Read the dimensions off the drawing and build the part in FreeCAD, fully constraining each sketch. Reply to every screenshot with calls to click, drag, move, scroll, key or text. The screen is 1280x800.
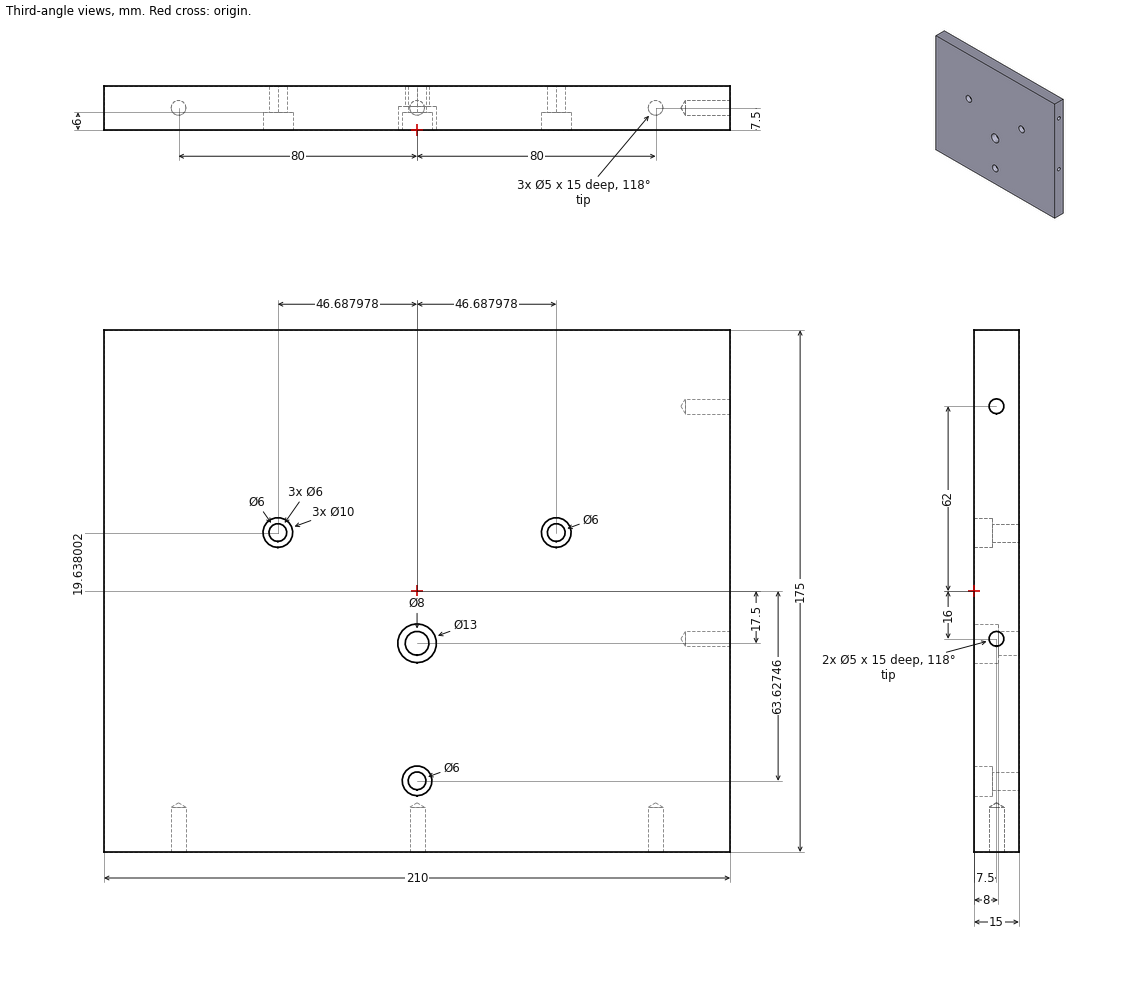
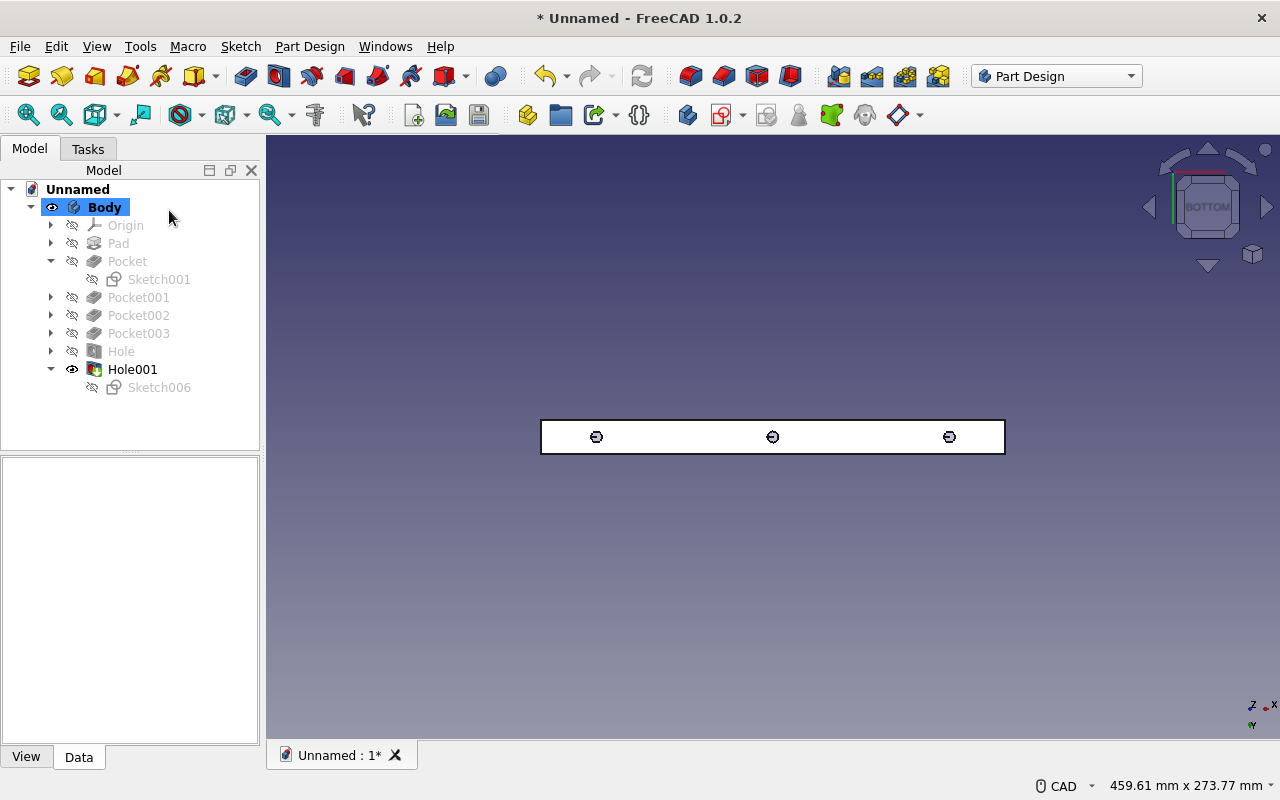
click(720, 116)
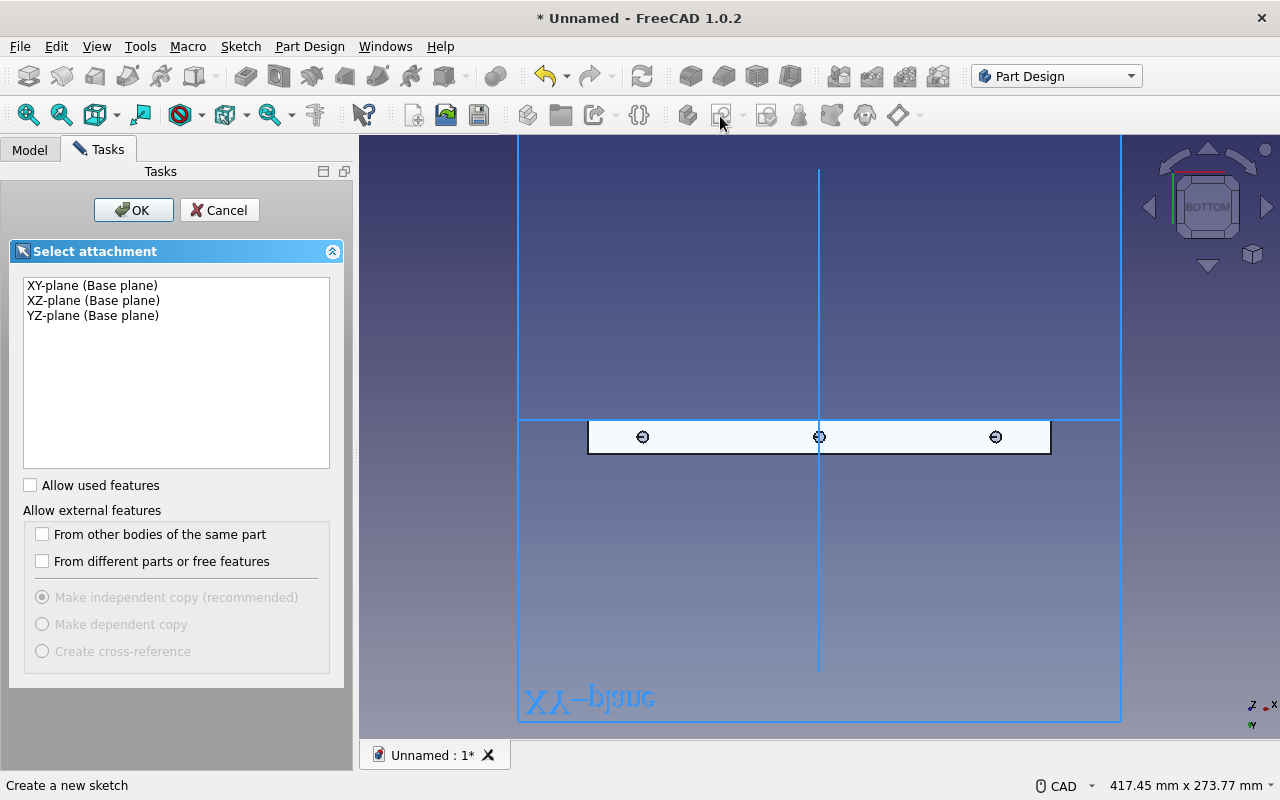
click(84, 300)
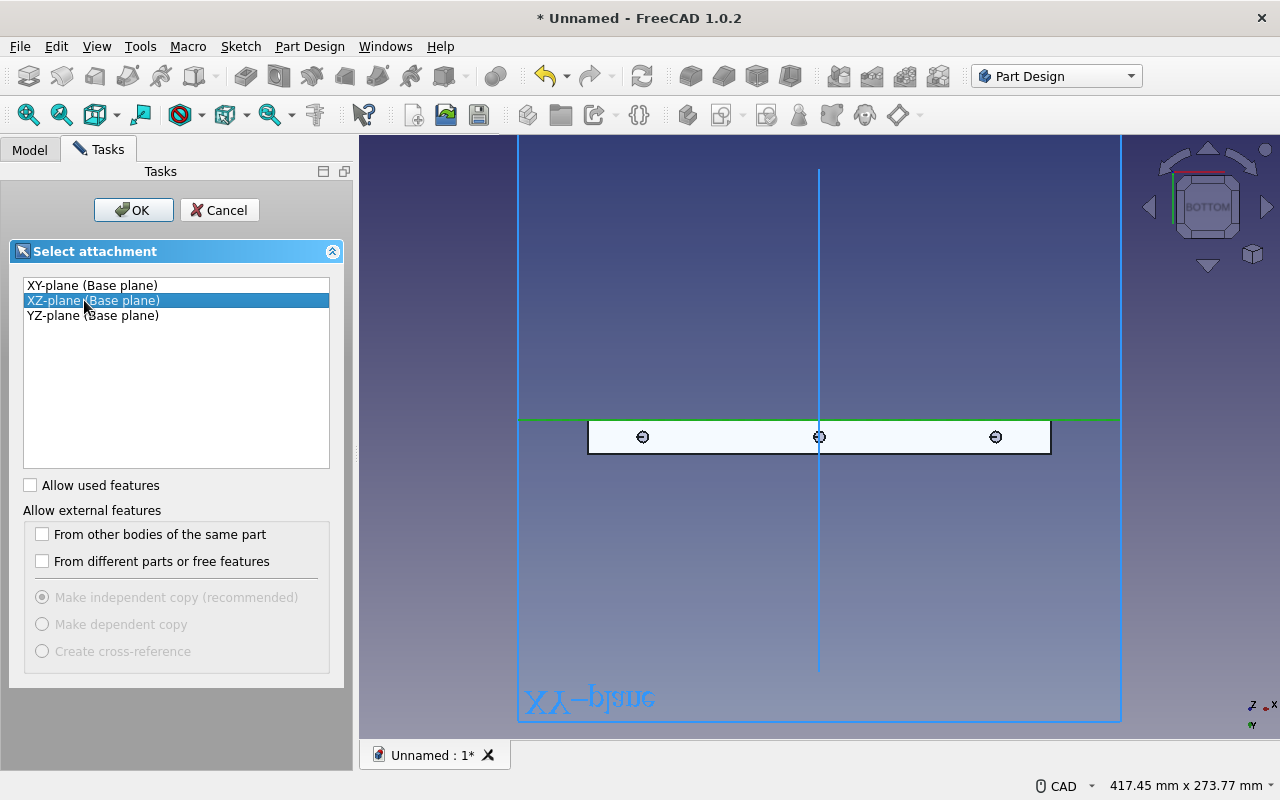
click(134, 210)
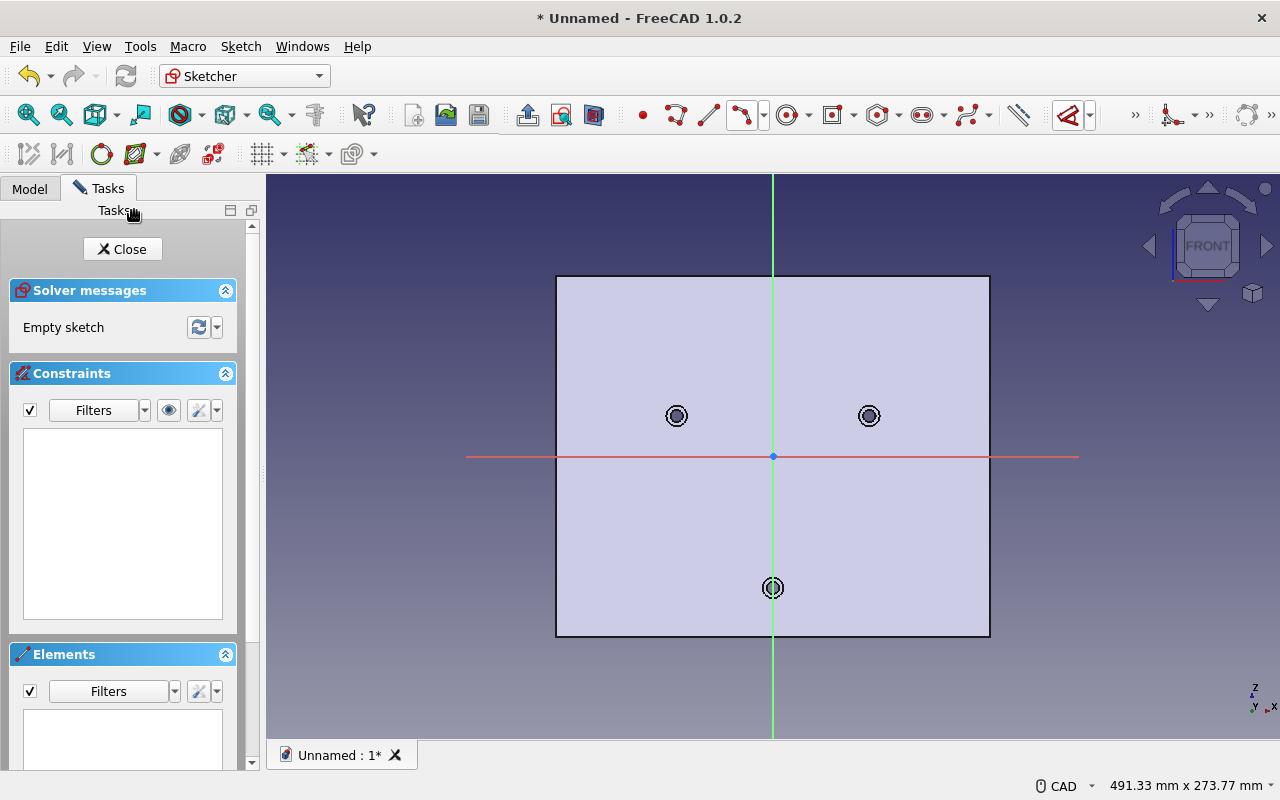
scroll(784, 485, up, 10)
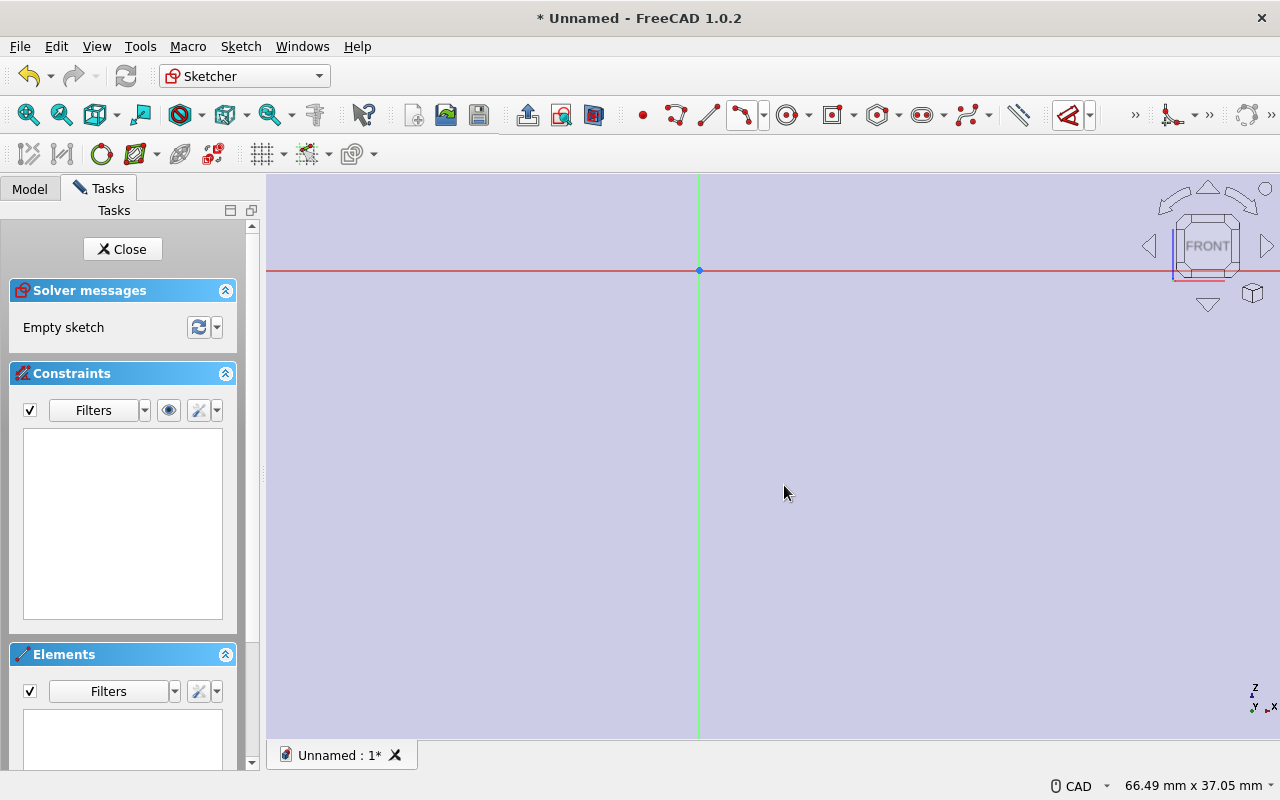
click(786, 116)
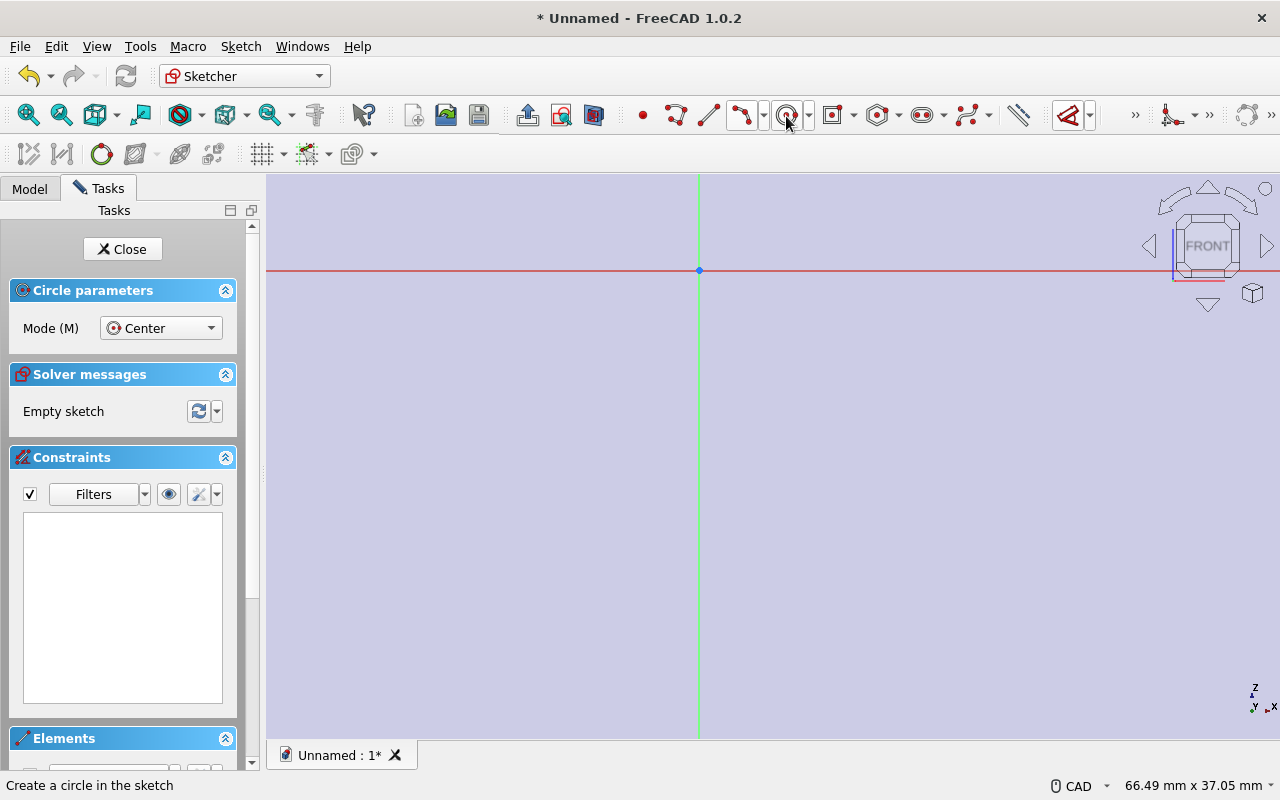
click(699, 538)
click(770, 468)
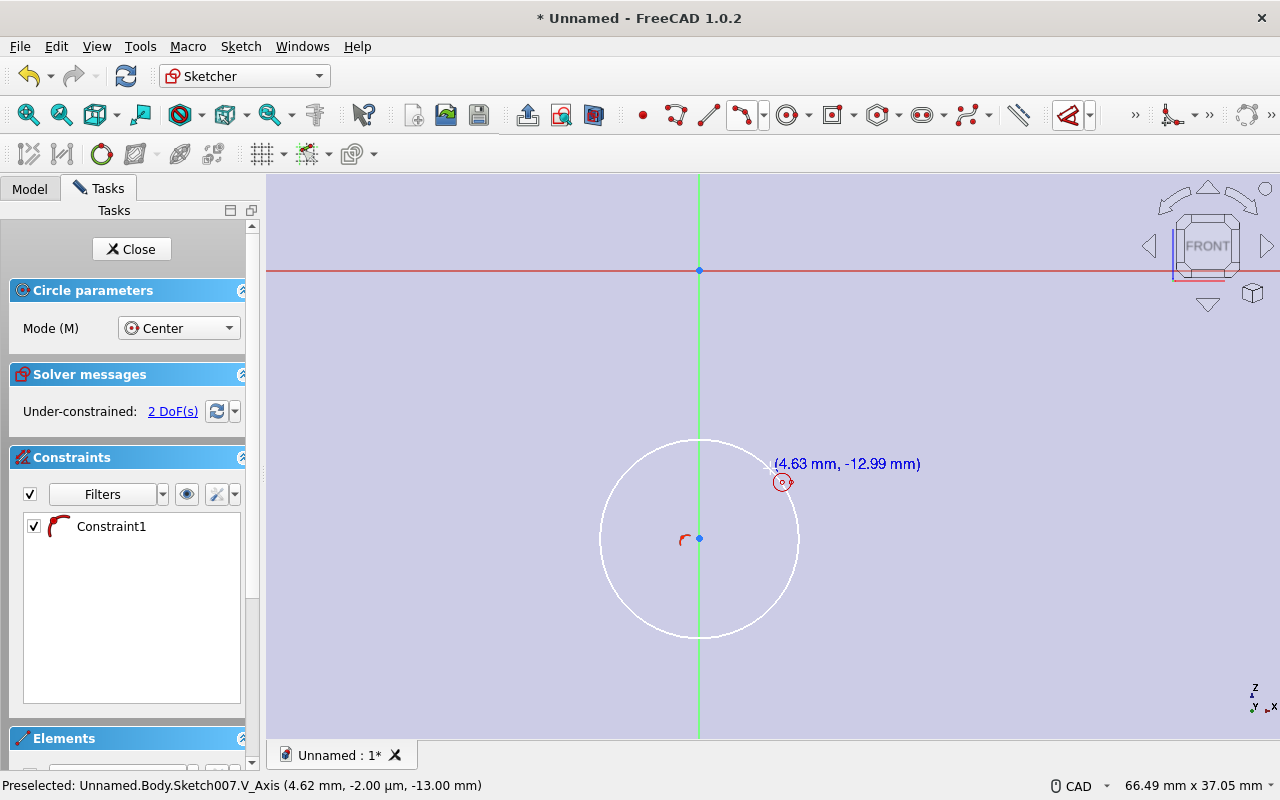
click(699, 539)
click(743, 495)
key(Escape)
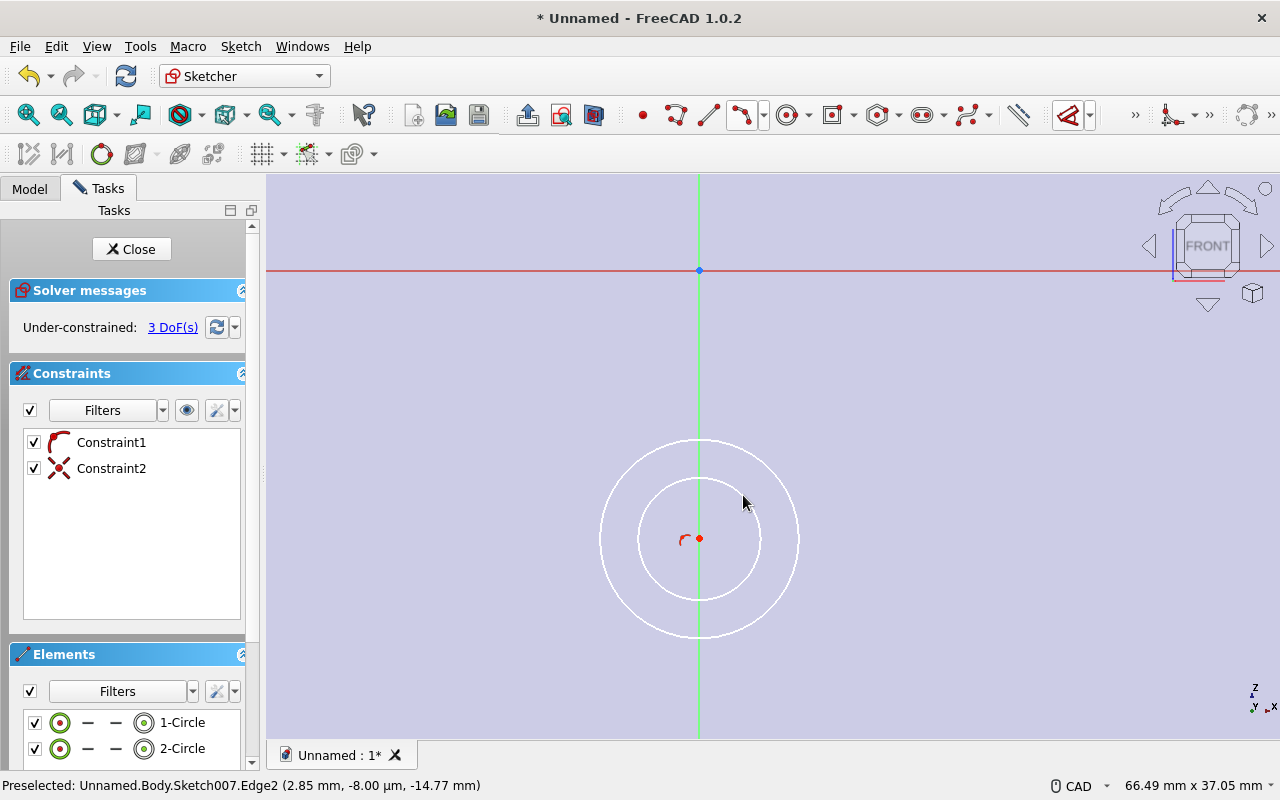
click(770, 469)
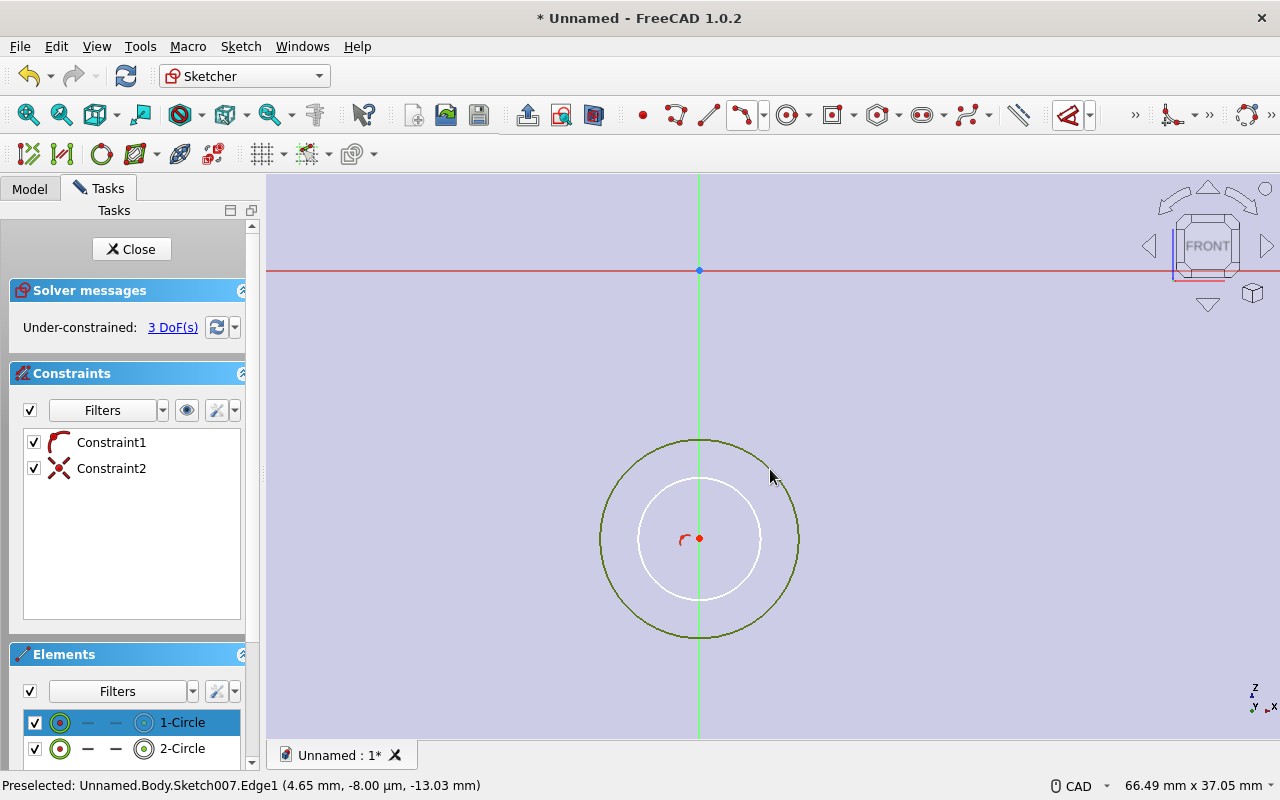
click(1090, 116)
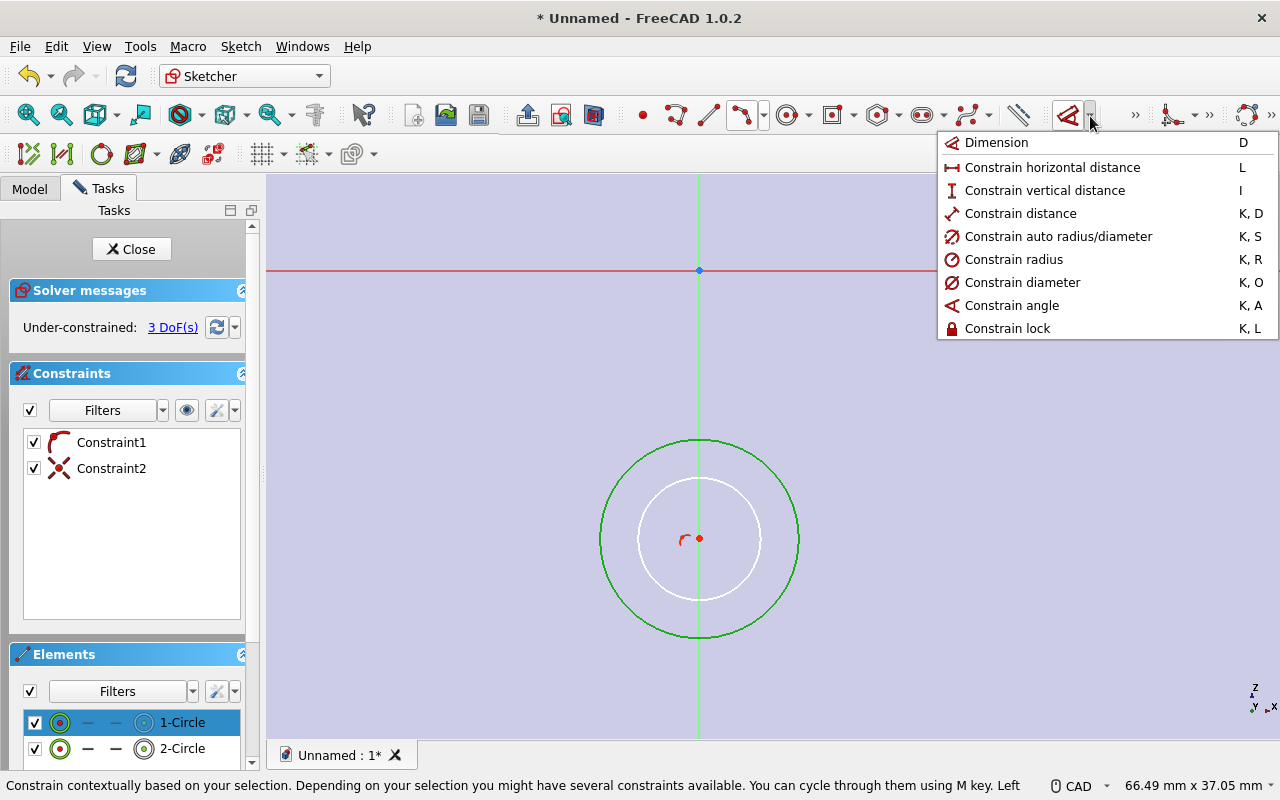
click(1108, 282)